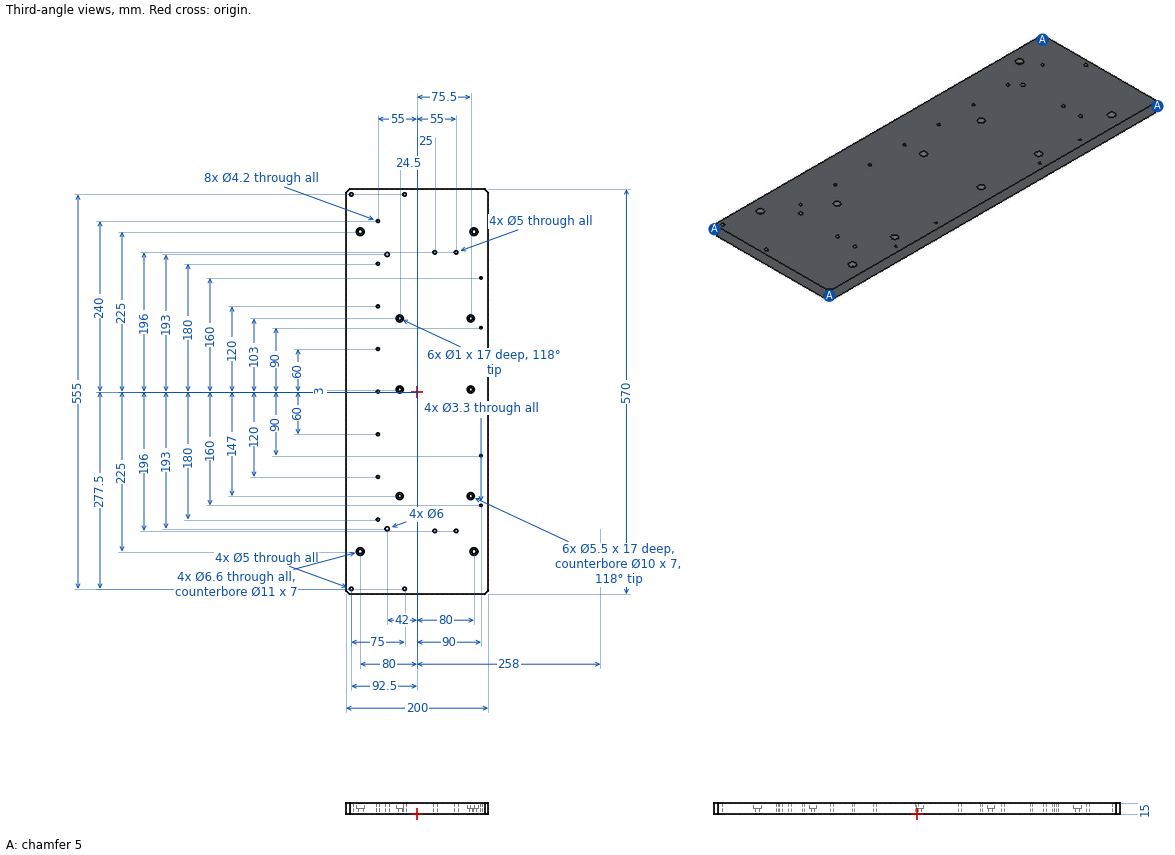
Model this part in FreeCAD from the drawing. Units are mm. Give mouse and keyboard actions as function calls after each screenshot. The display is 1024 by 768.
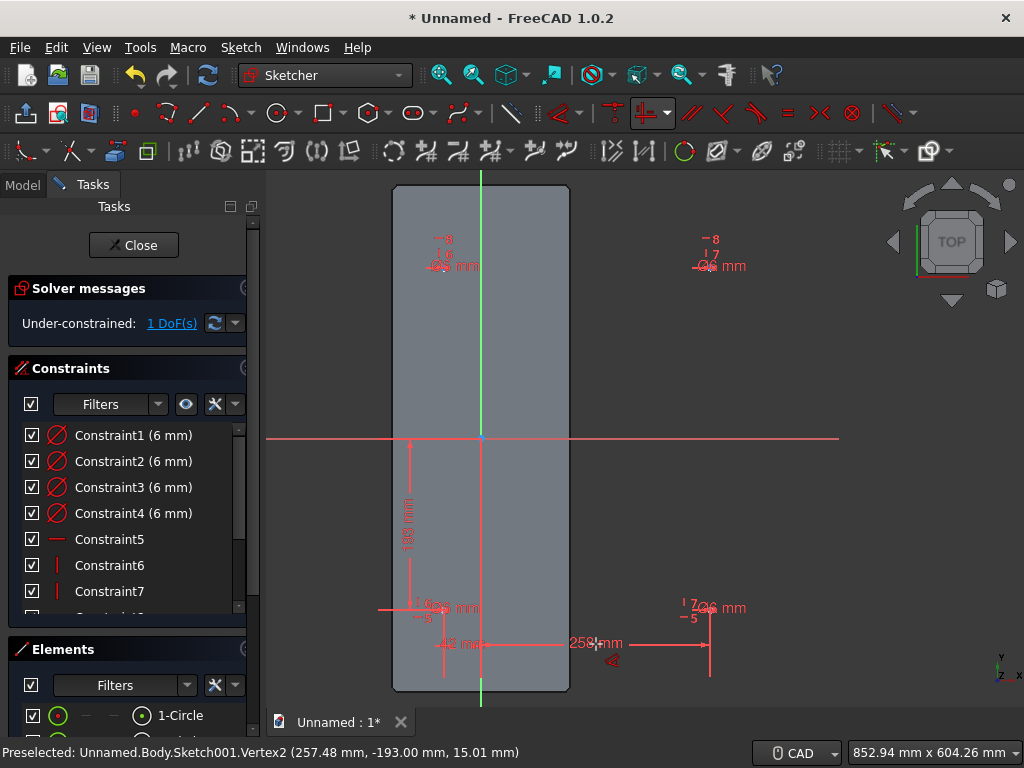
click(444, 268)
click(410, 353)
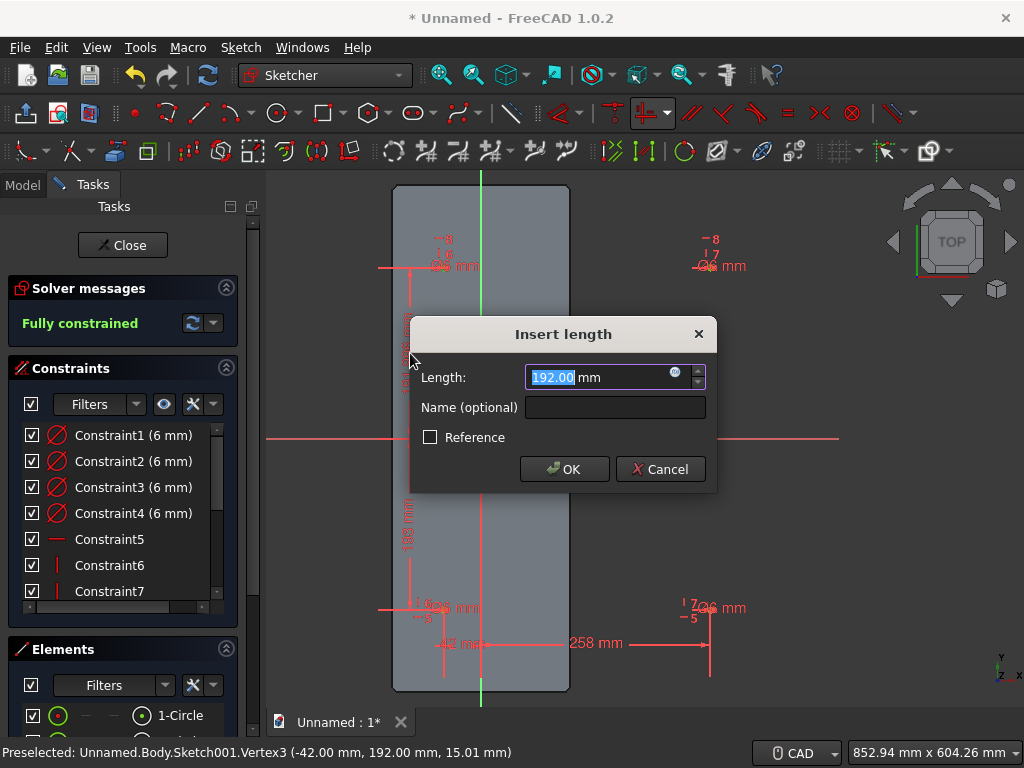
text(193)
key(Return)
key(Escape)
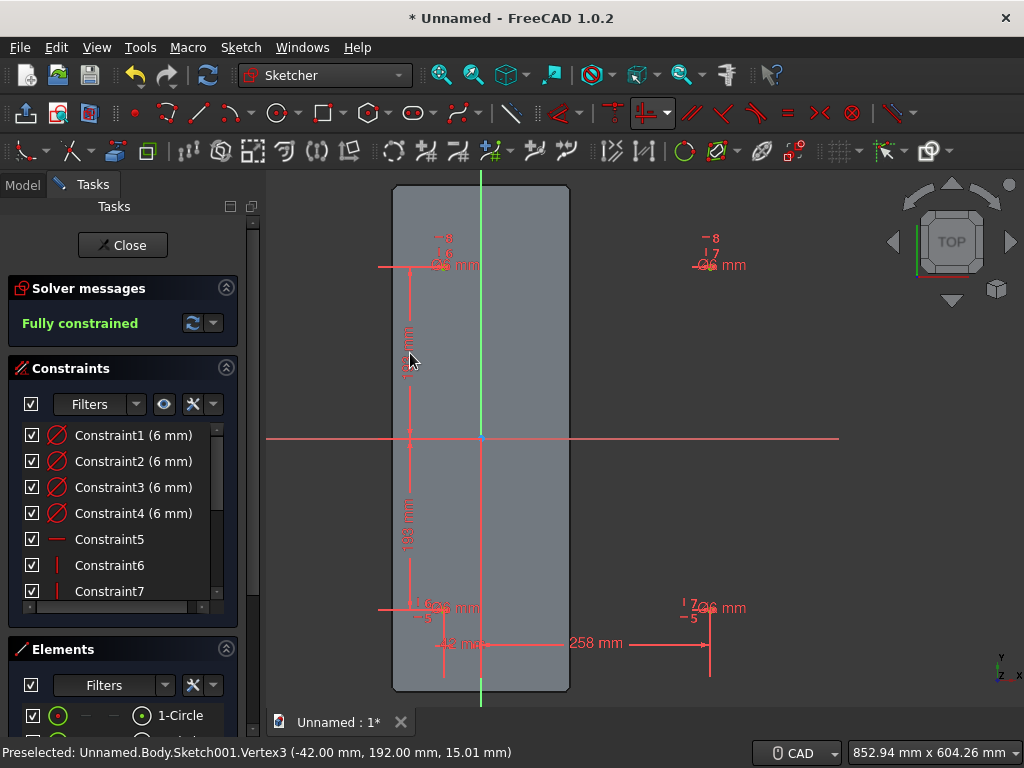
click(123, 245)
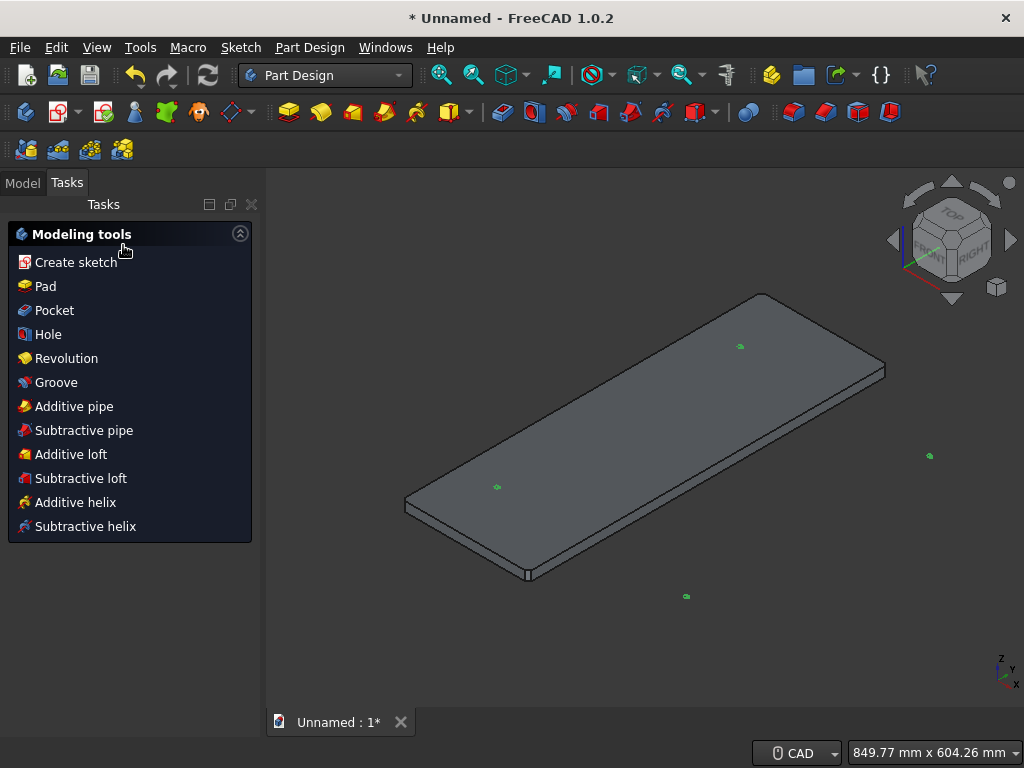
click(504, 112)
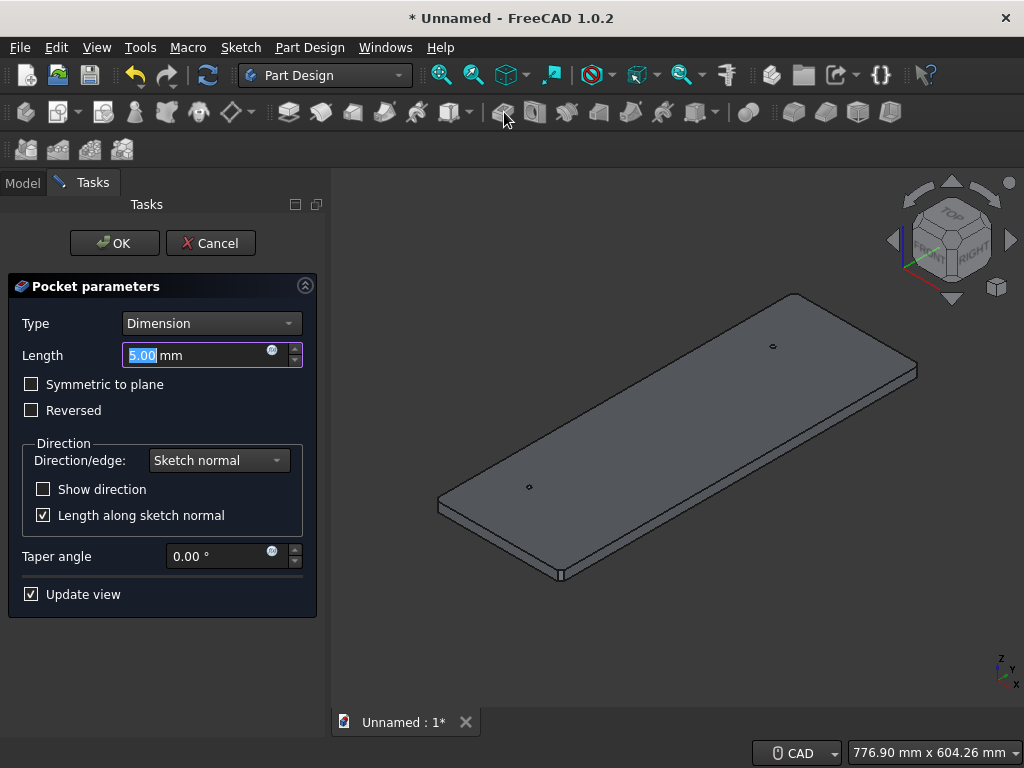
click(212, 324)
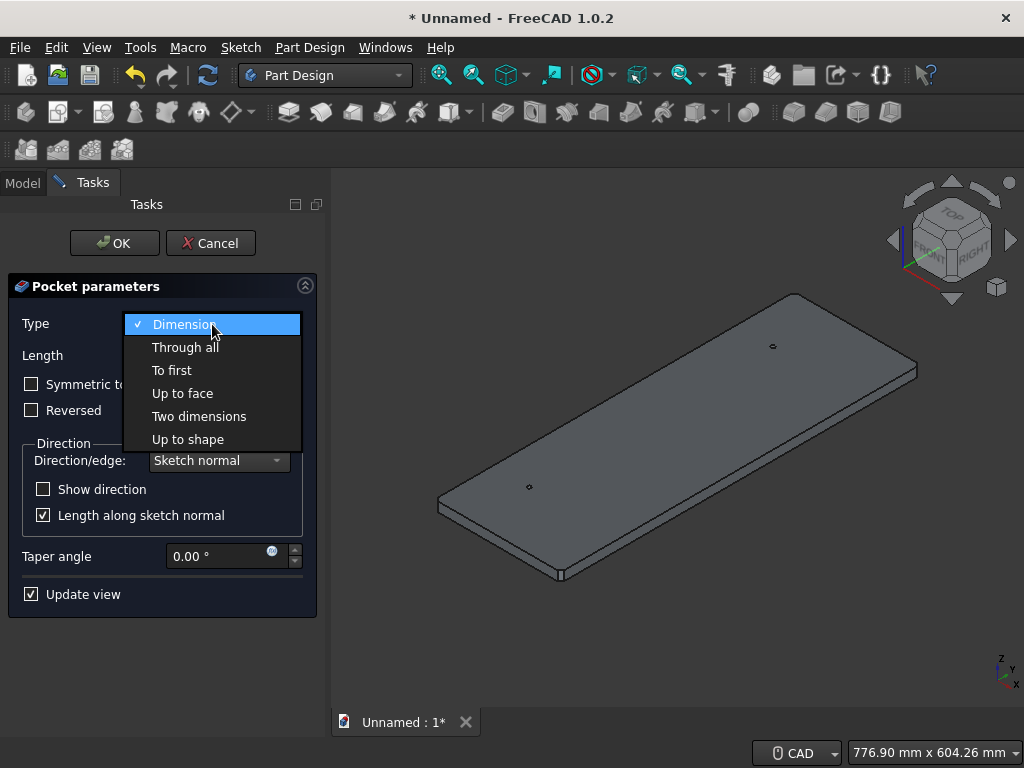
click(212, 348)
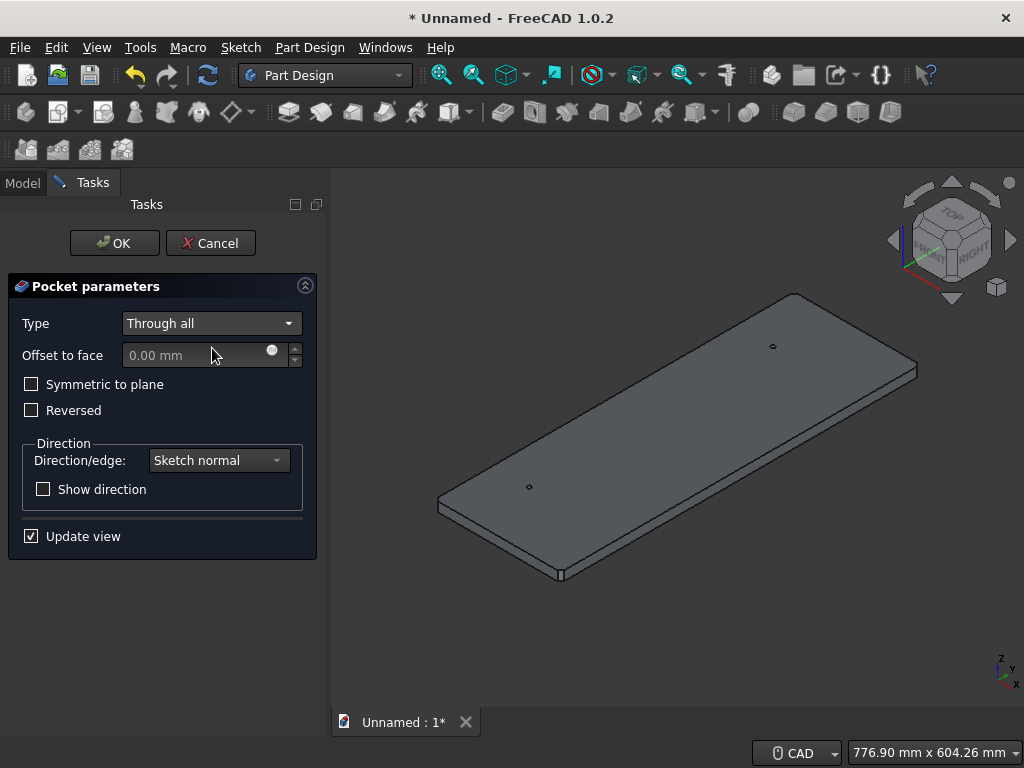
click(115, 243)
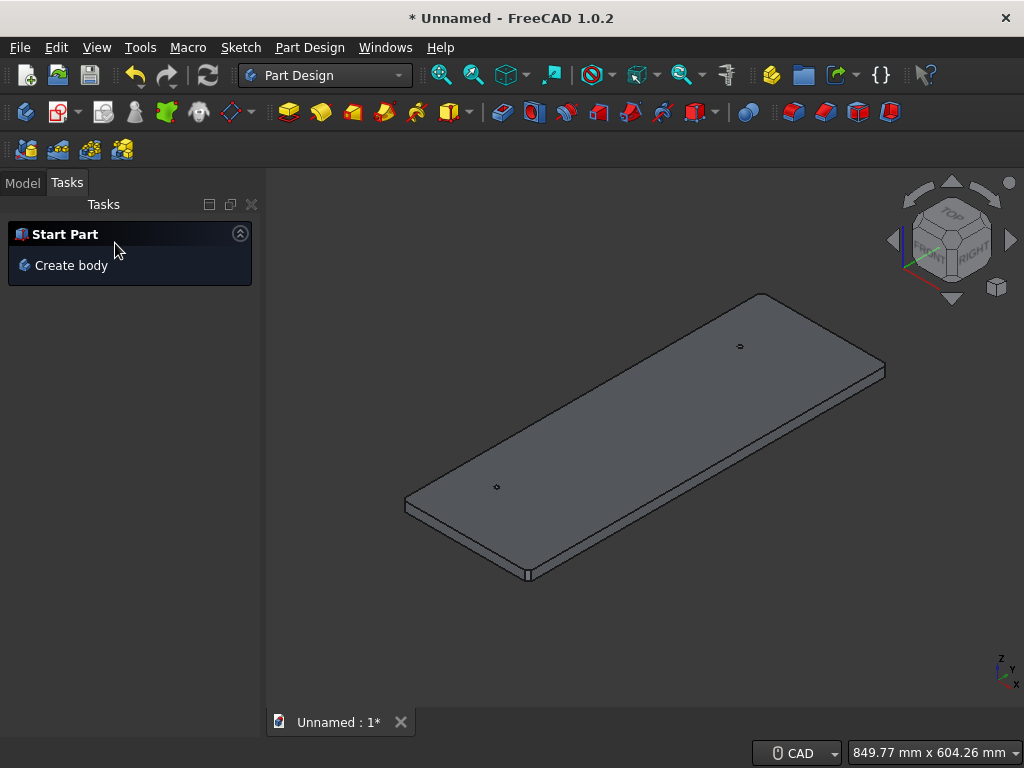
click(696, 401)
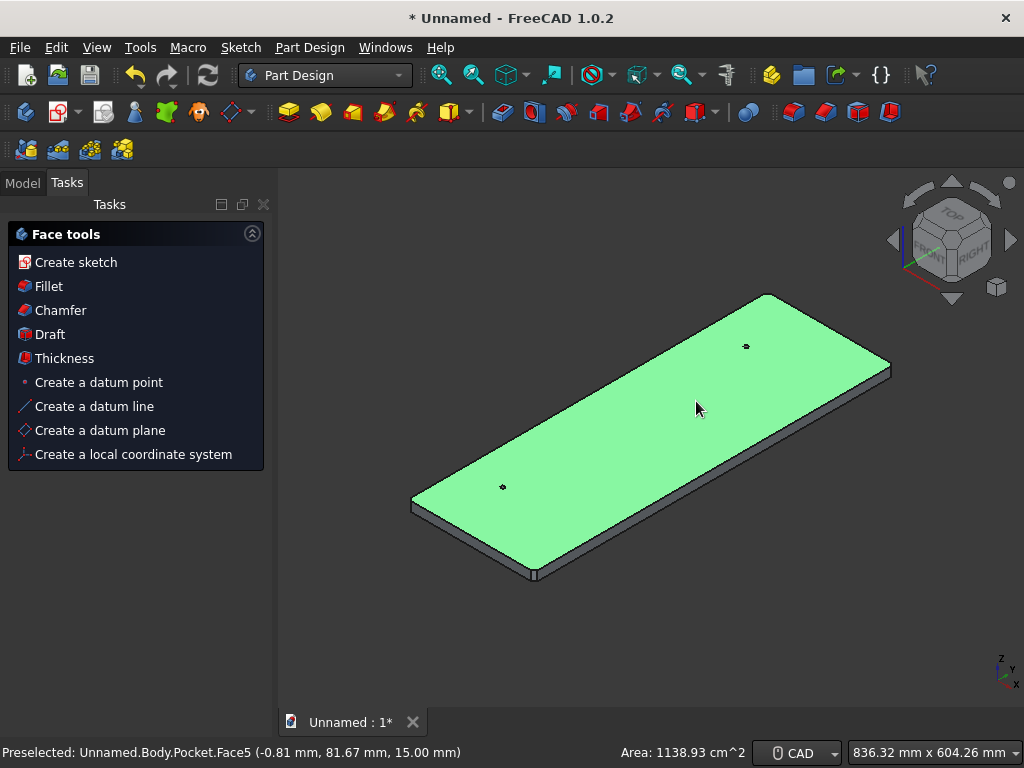
click(58, 112)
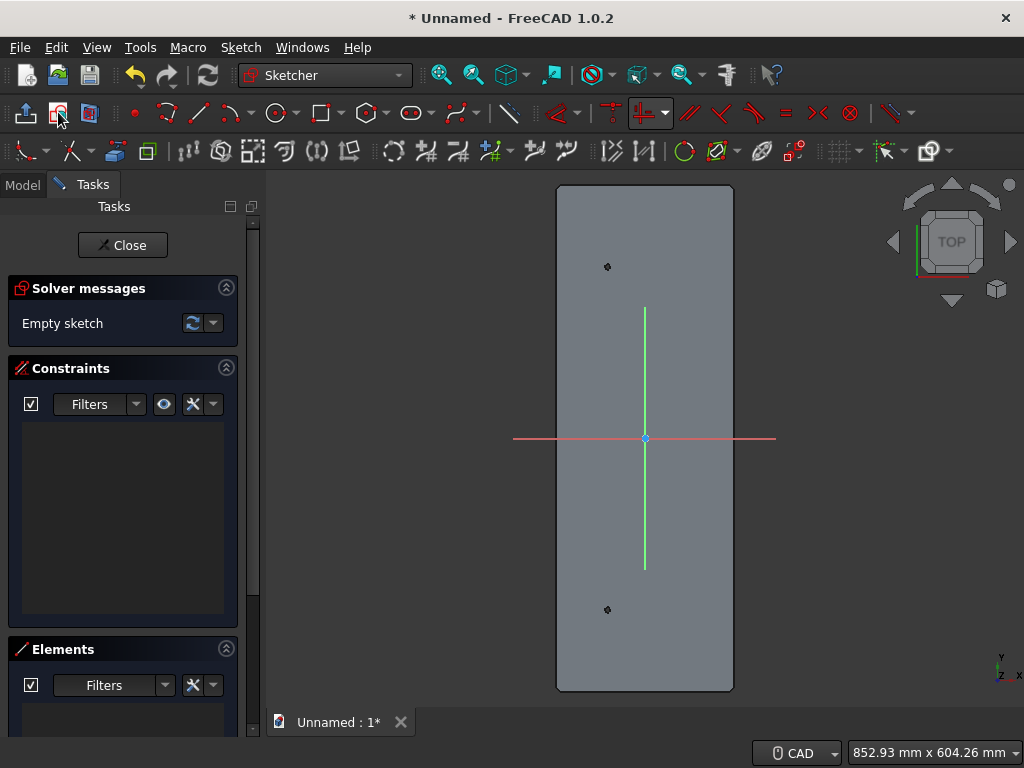
click(276, 114)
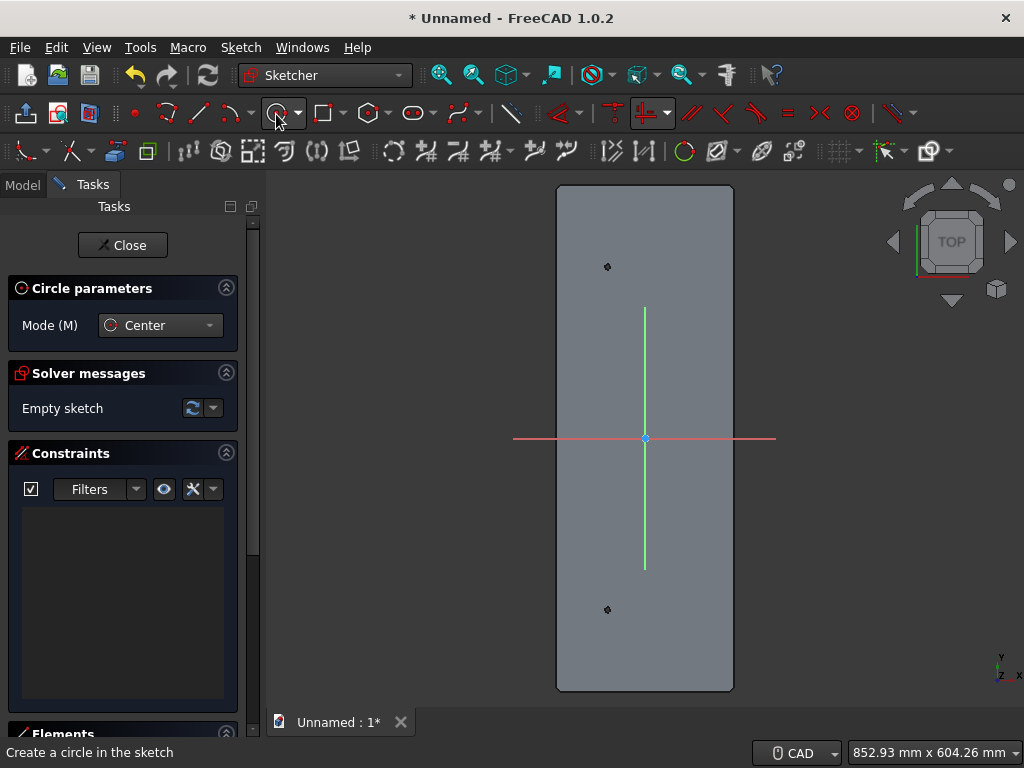
scroll(694, 264, up, 12)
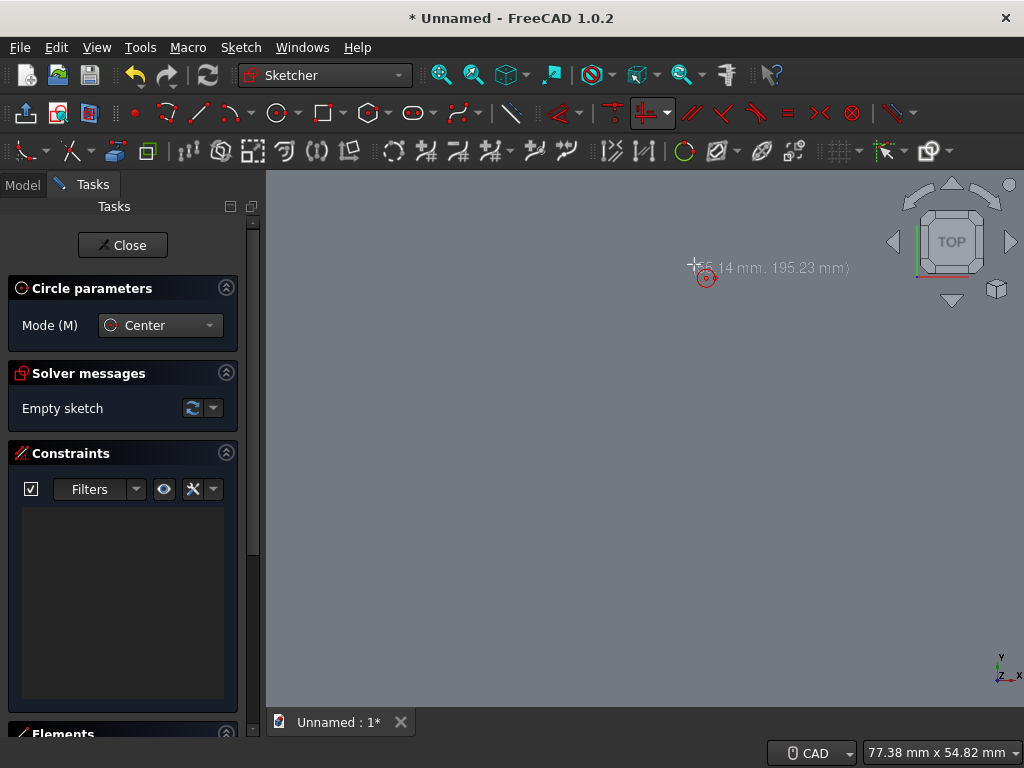
scroll(591, 264, down, 12)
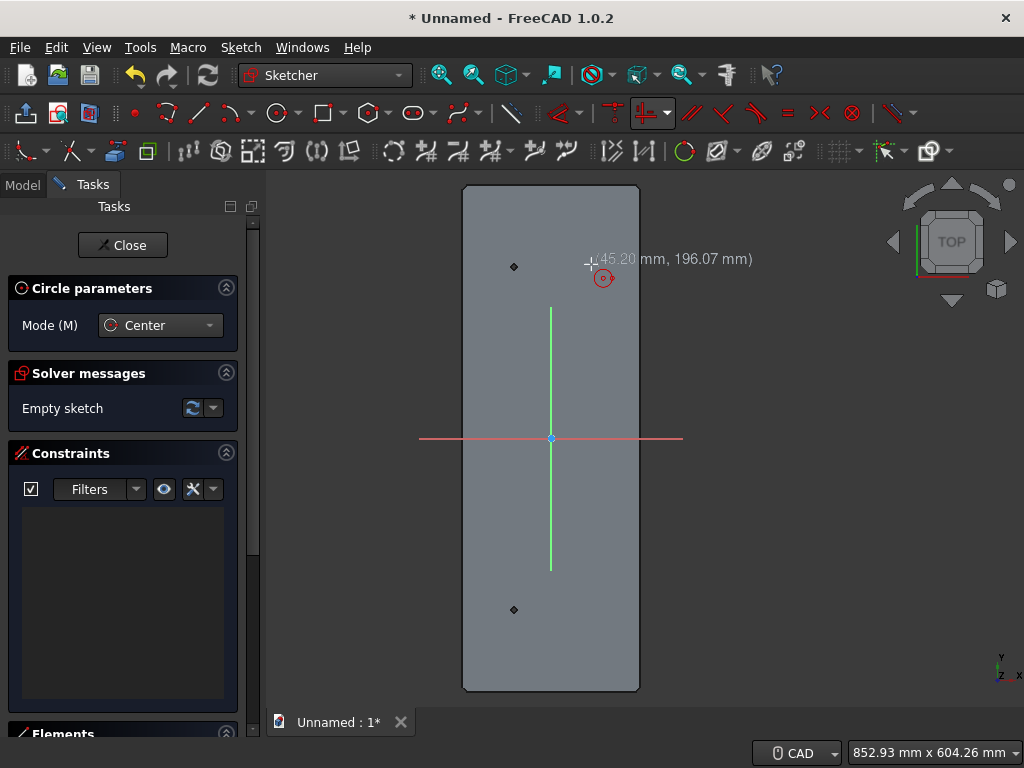
click(600, 264)
move(602, 263)